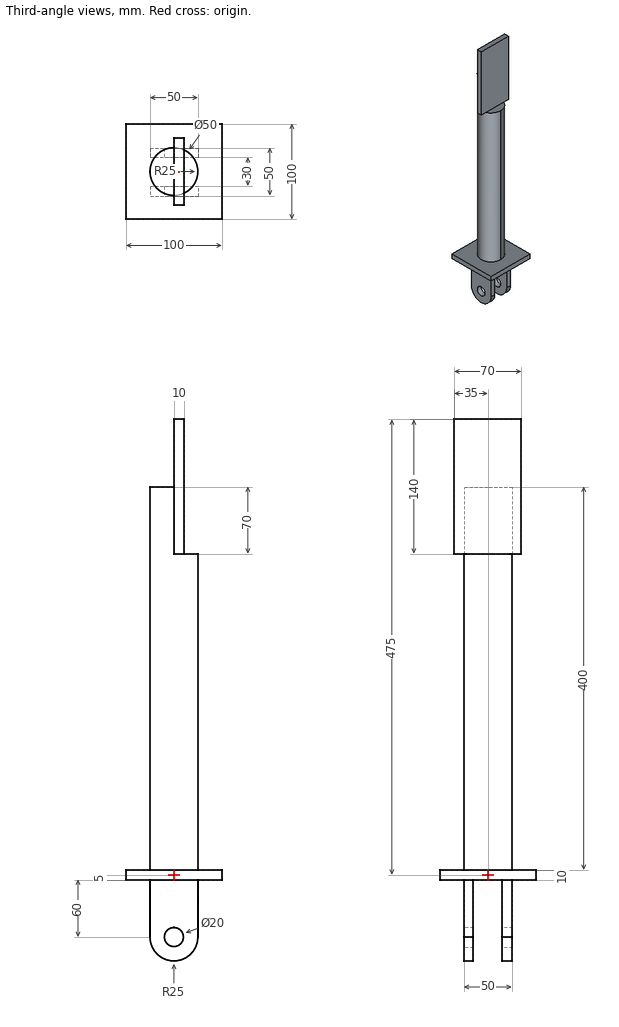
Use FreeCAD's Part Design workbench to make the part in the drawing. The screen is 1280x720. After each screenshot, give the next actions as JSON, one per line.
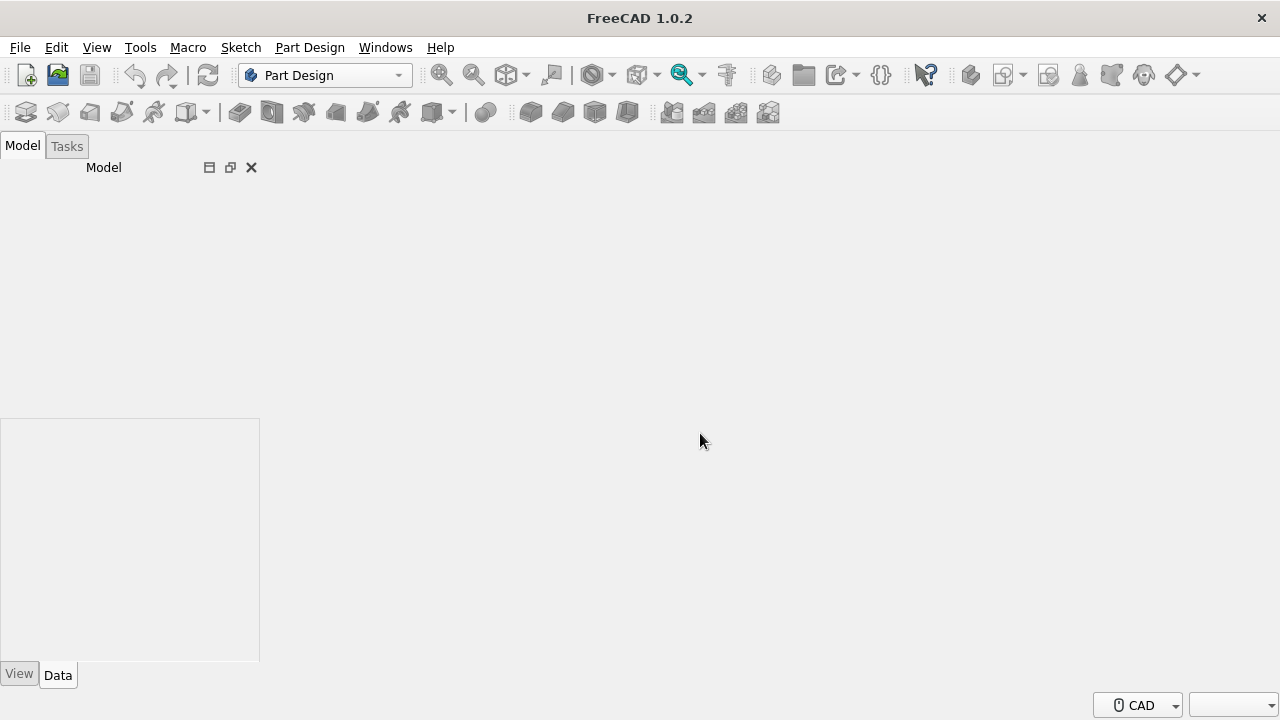
{"action": "key", "text": "ctrl+n"}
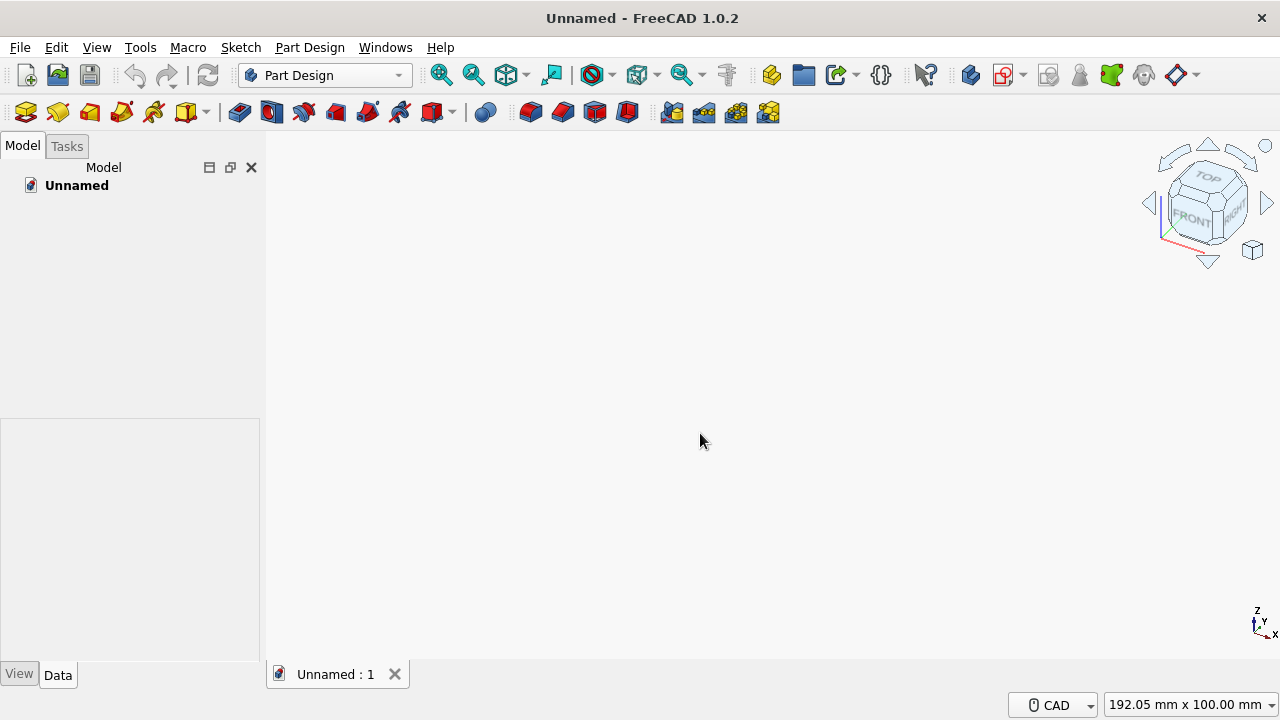
{"action": "left_click", "coordinate": [1004, 76]}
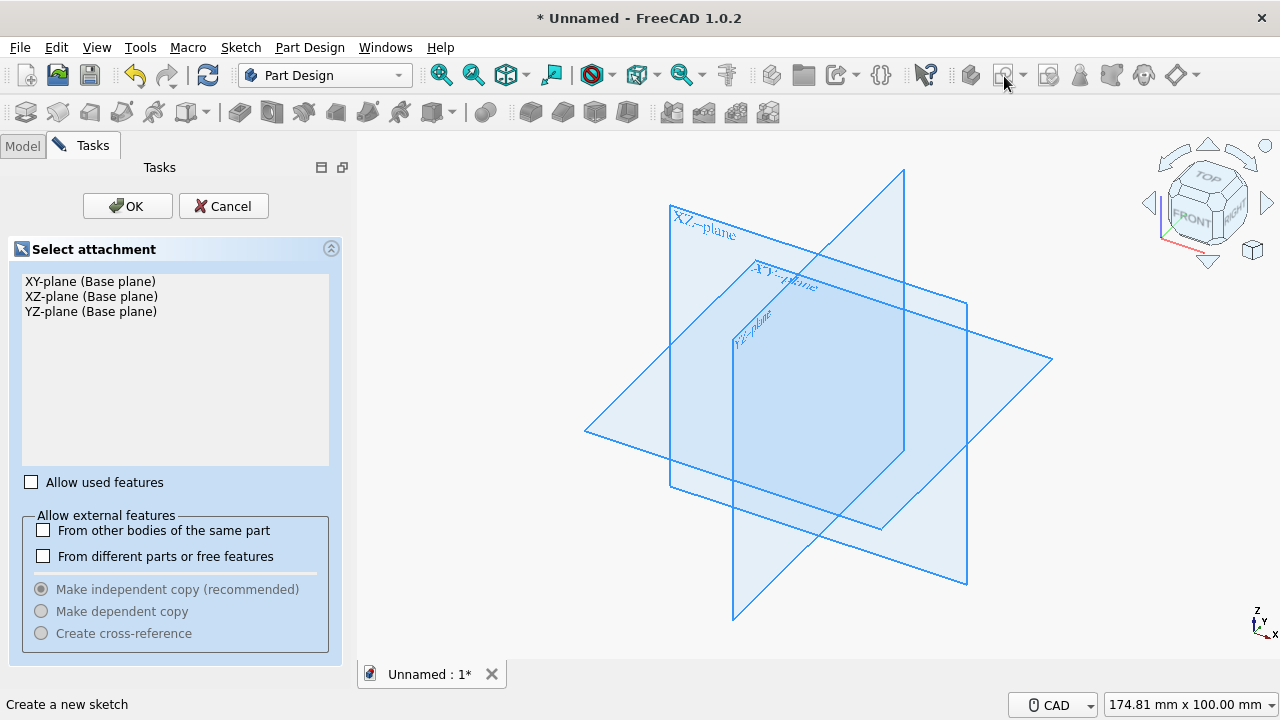
{"action": "left_click", "coordinate": [82, 282]}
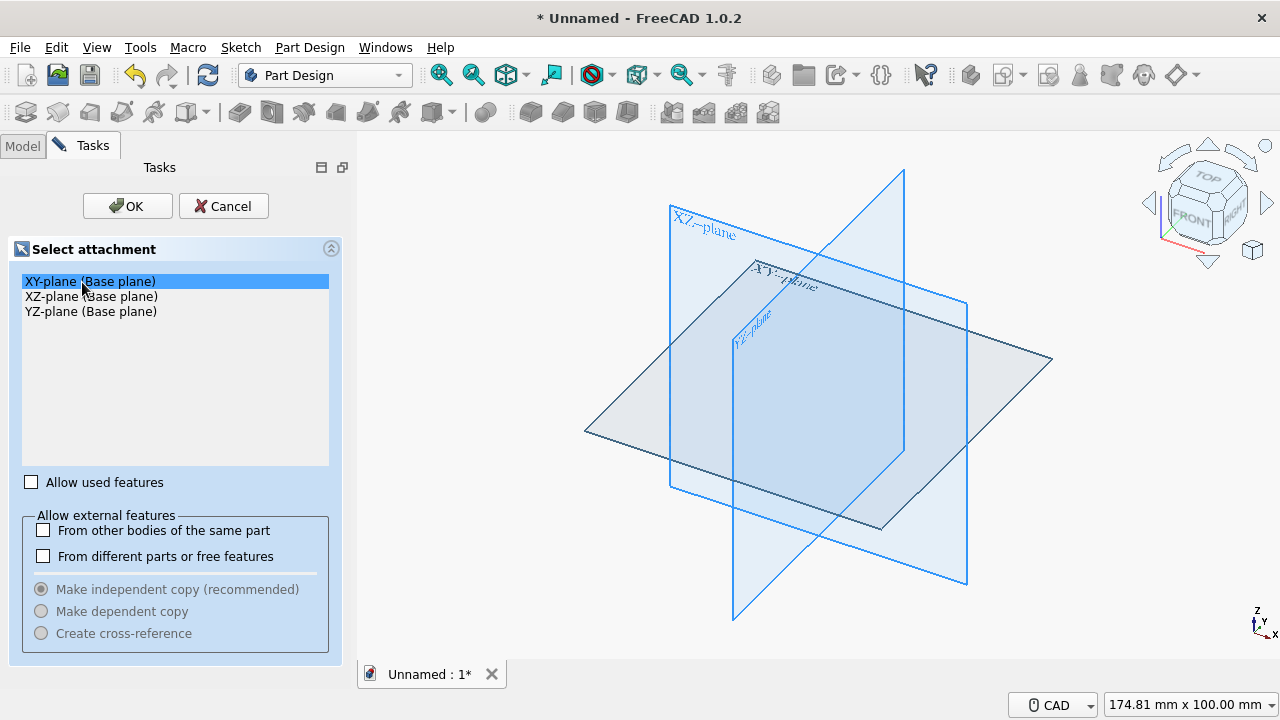
{"action": "left_click", "coordinate": [128, 206]}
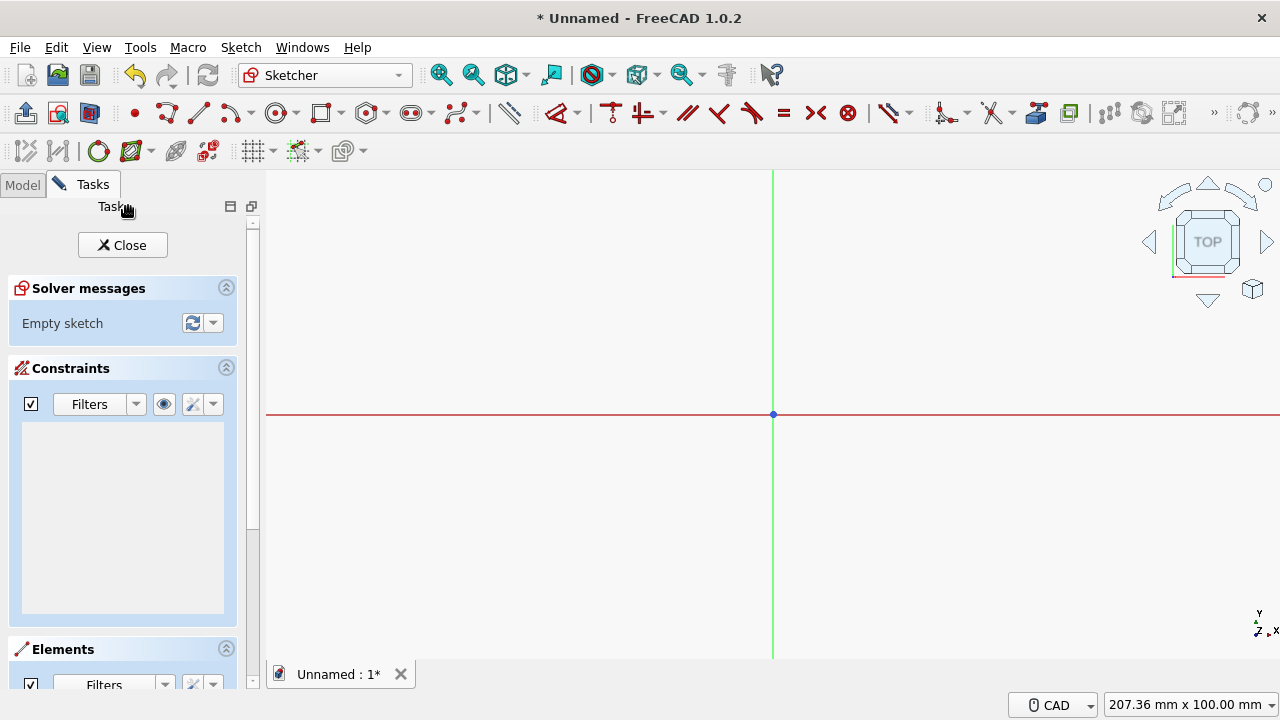
{"action": "scroll", "coordinate": [565, 414], "scroll_direction": "down", "scroll_amount": 2}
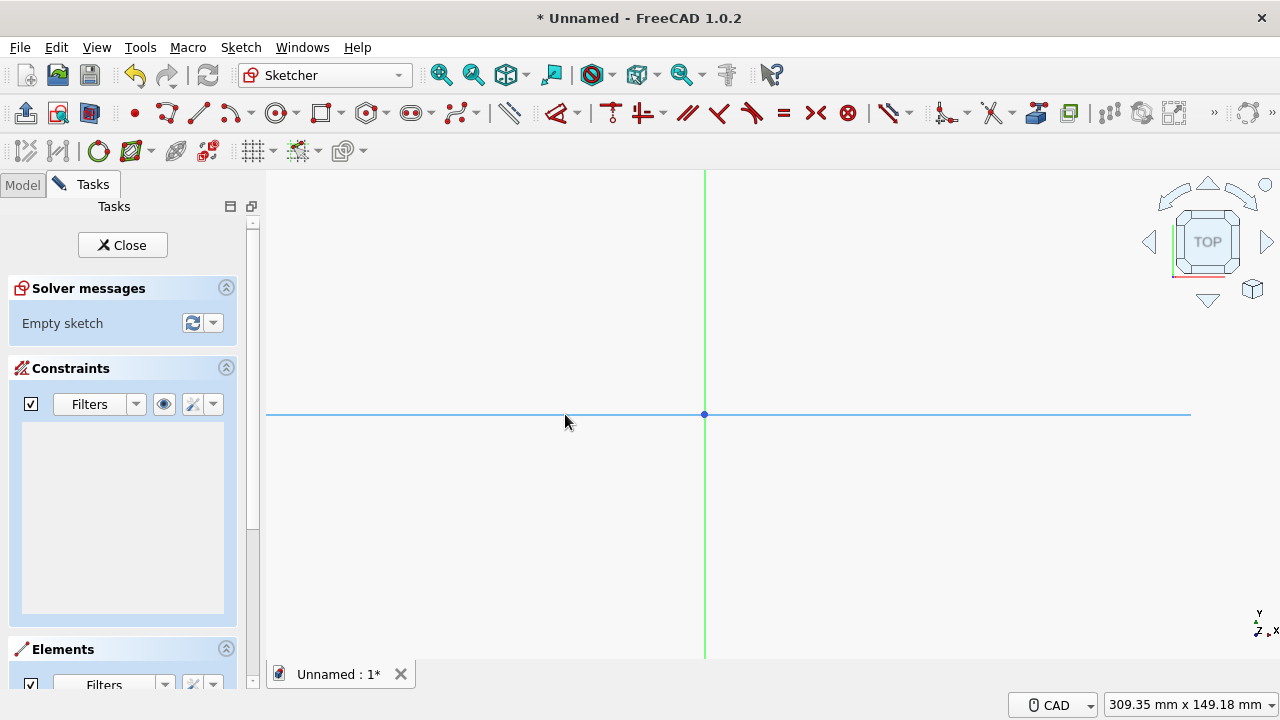
{"action": "key", "text": "g v"}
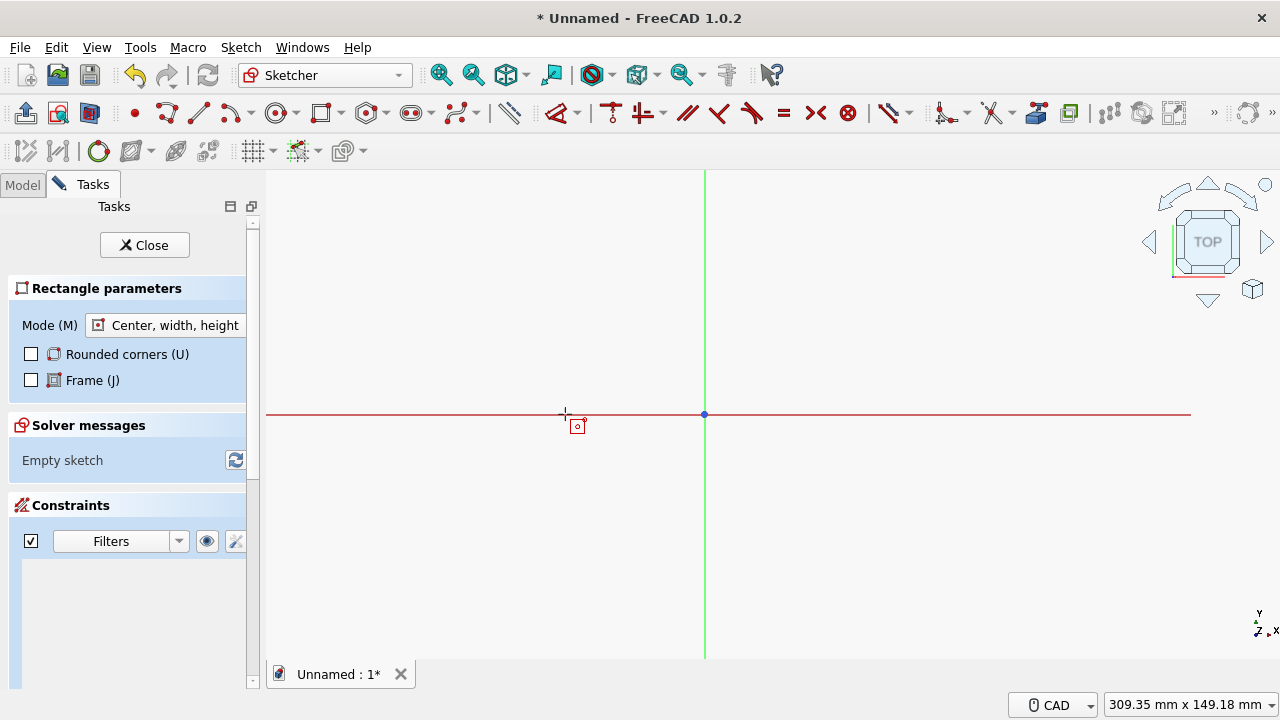
{"action": "left_click", "coordinate": [705, 414]}
{"action": "left_click", "coordinate": [868, 251]}
{"action": "key", "text": "Escape"}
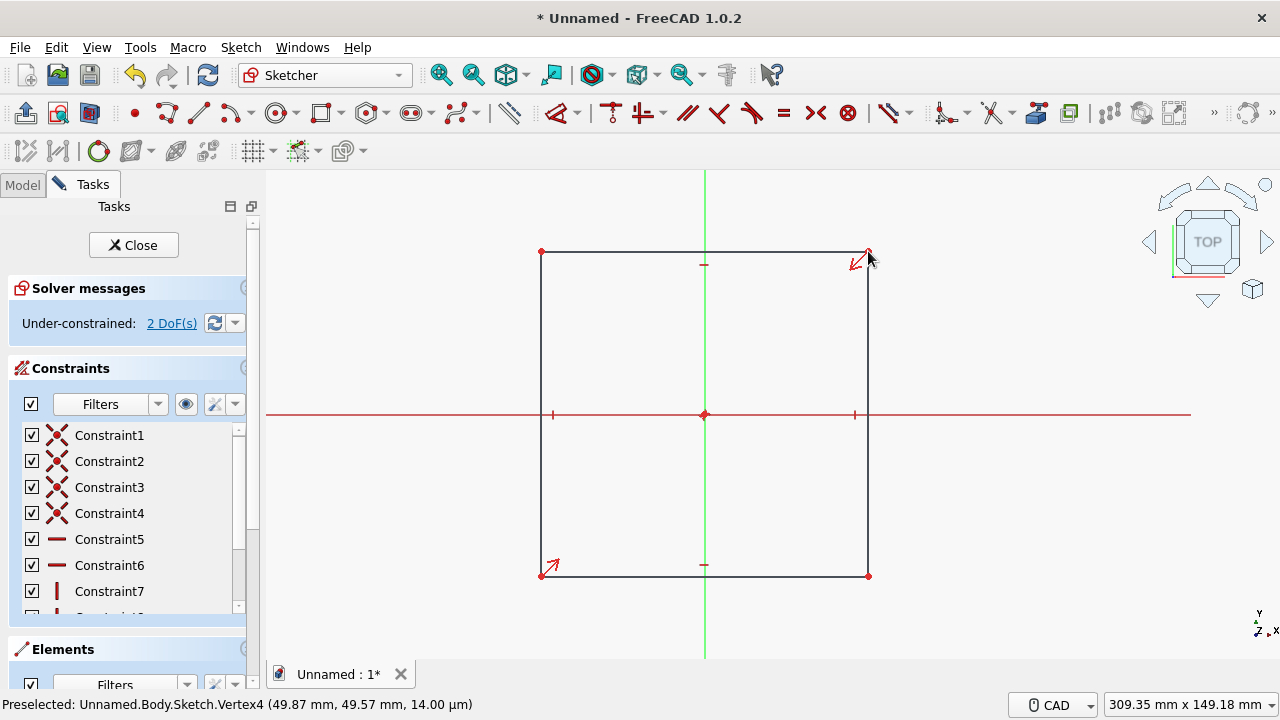
{"action": "key", "text": "d"}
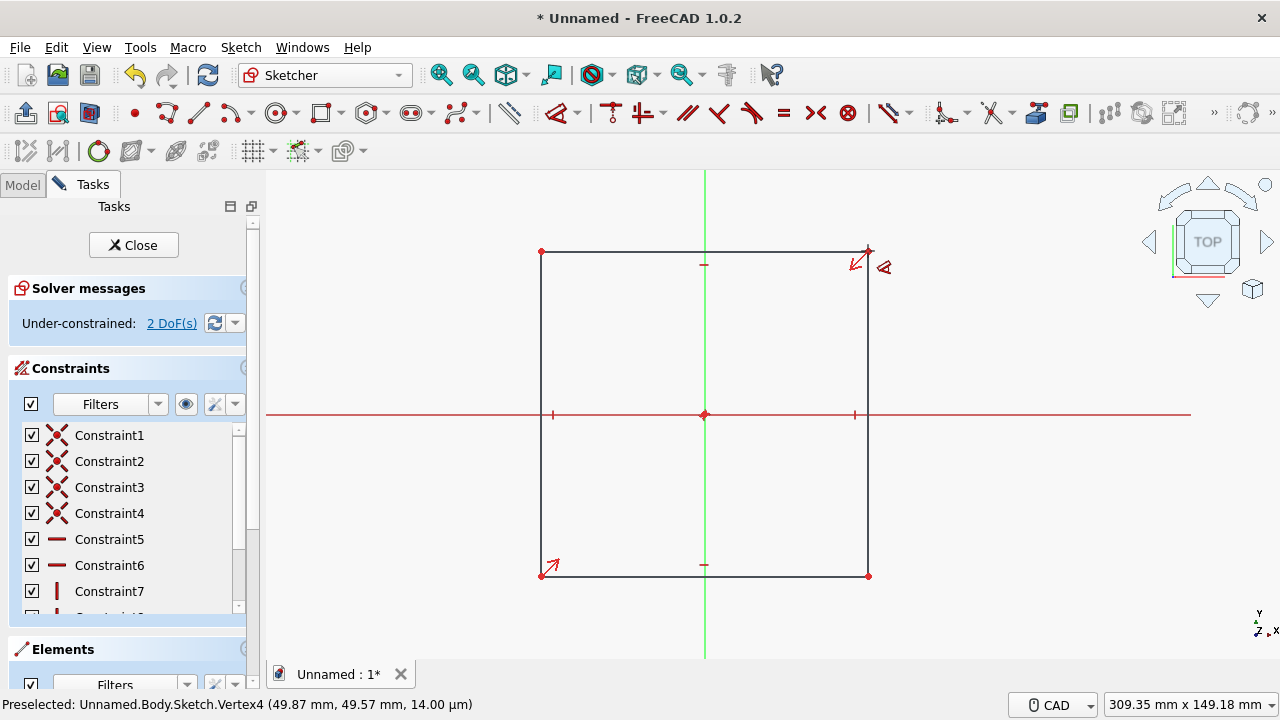
{"action": "left_click", "coordinate": [639, 577]}
{"action": "left_click", "coordinate": [629, 611]}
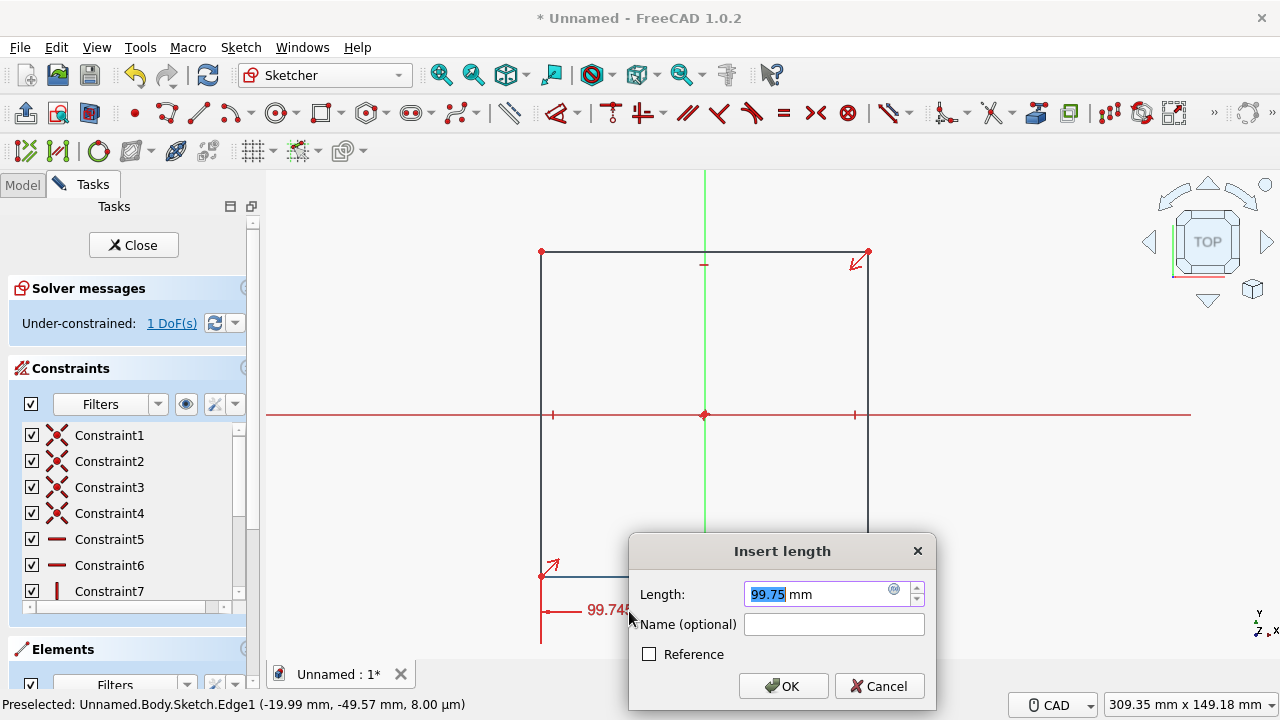
{"action": "type", "text": "100"}
{"action": "key", "text": "Return"}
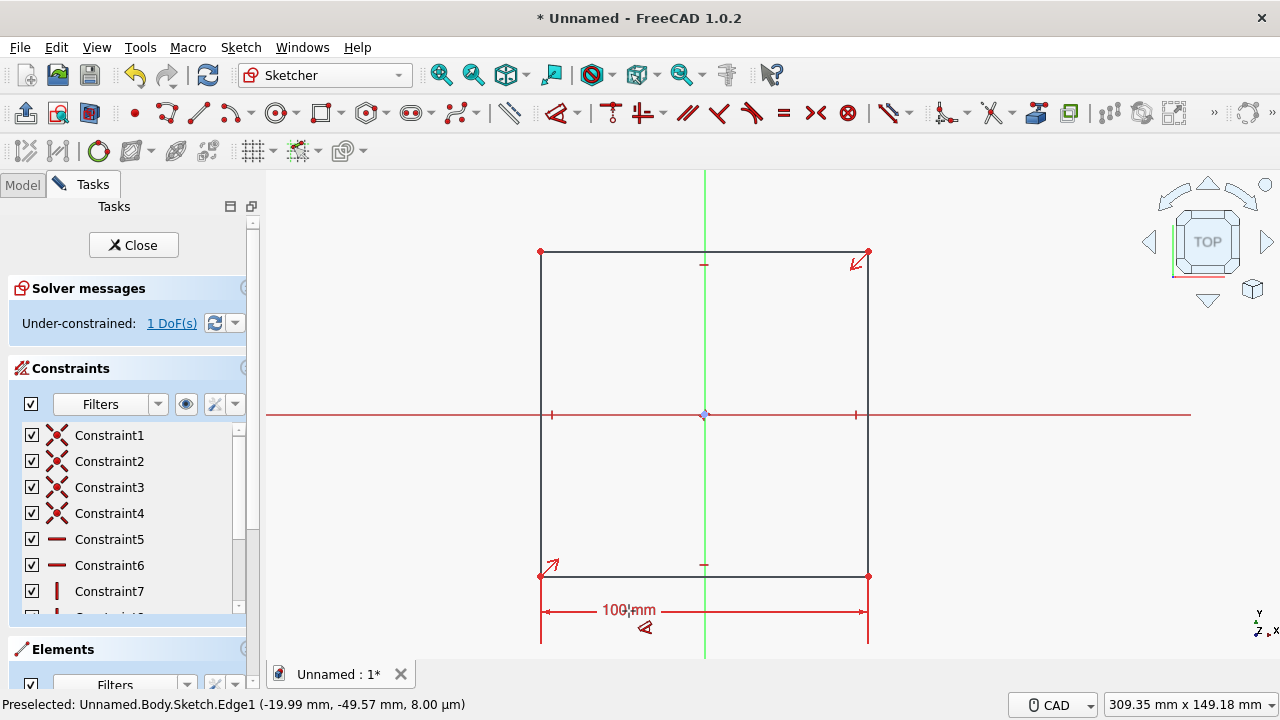
{"action": "left_click", "coordinate": [868, 480]}
{"action": "left_click", "coordinate": [902, 340]}